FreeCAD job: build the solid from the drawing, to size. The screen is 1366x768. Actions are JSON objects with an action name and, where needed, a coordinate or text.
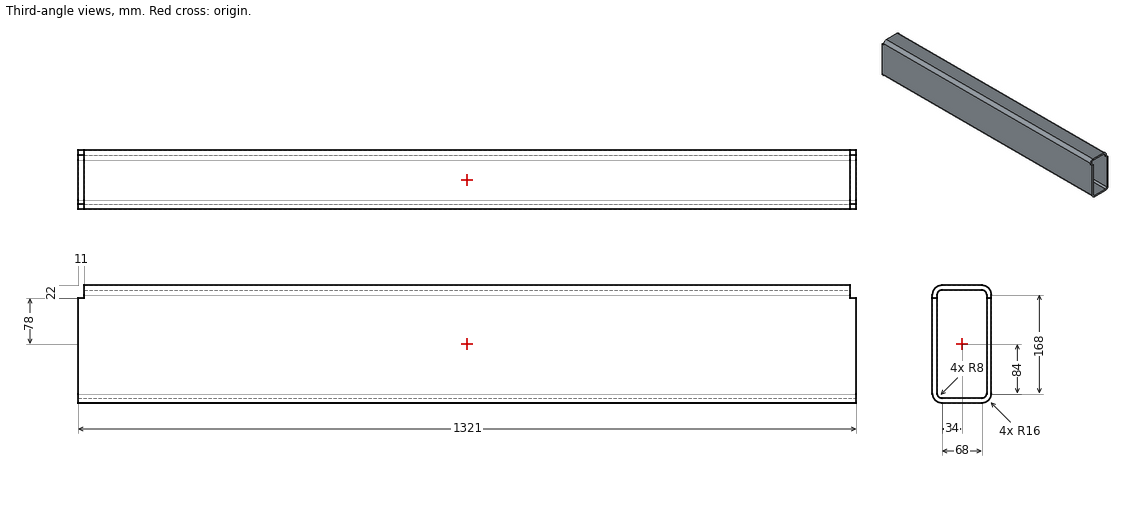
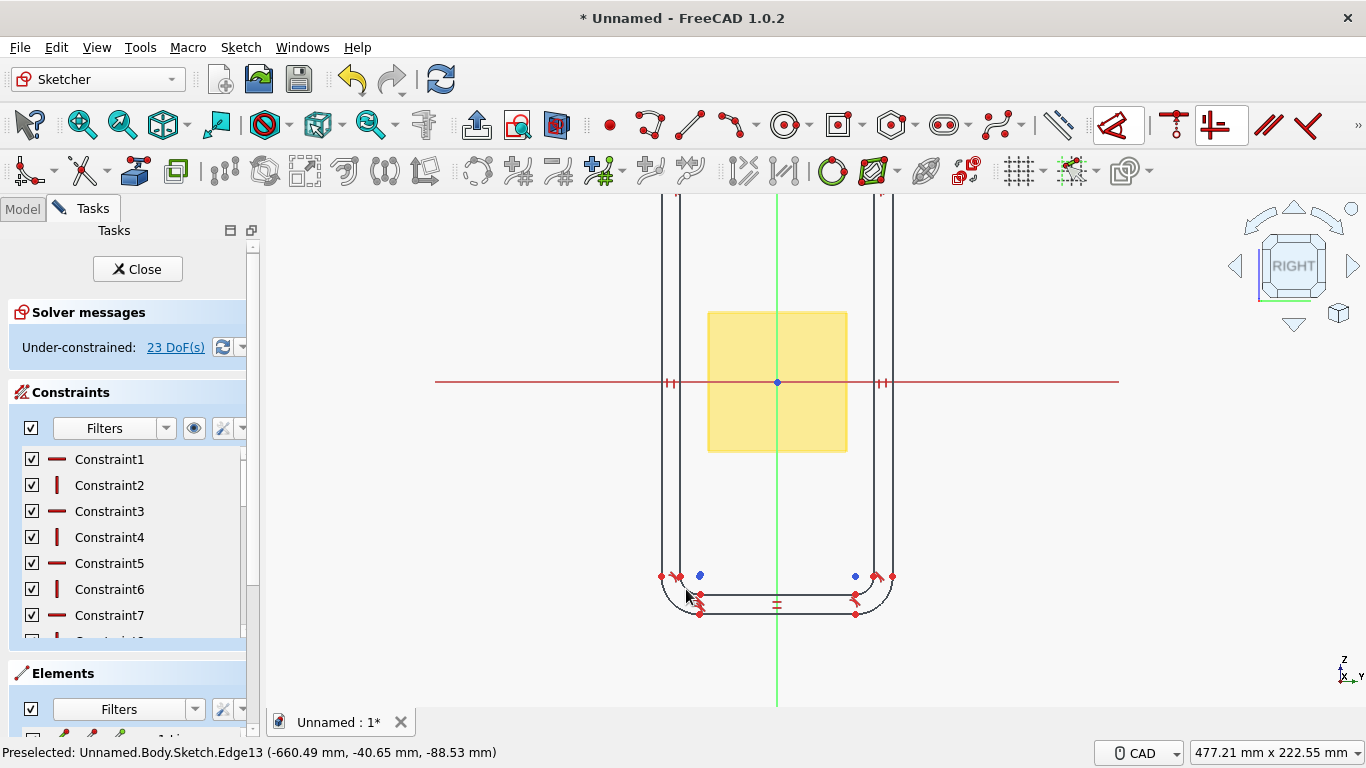
{"action": "left_click", "coordinate": [809, 595]}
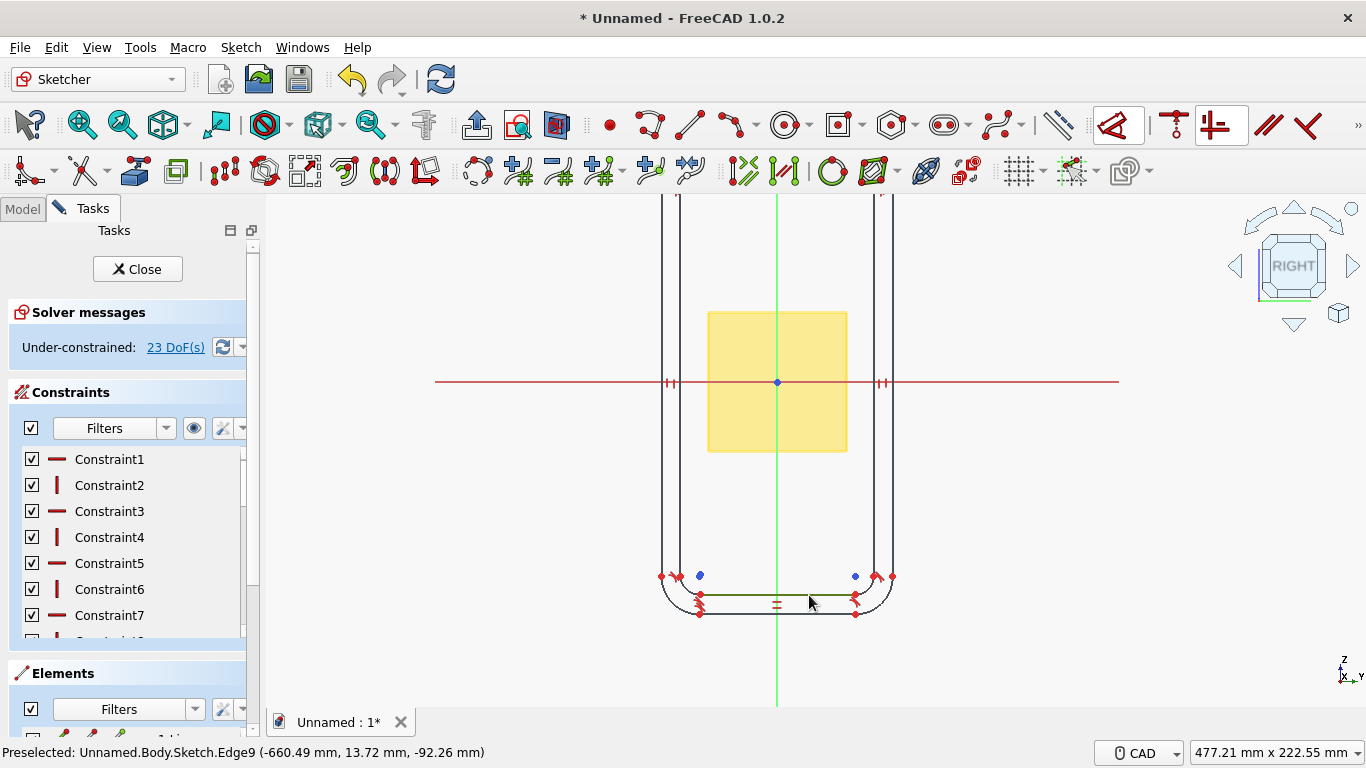
{"action": "left_click", "coordinate": [869, 589]}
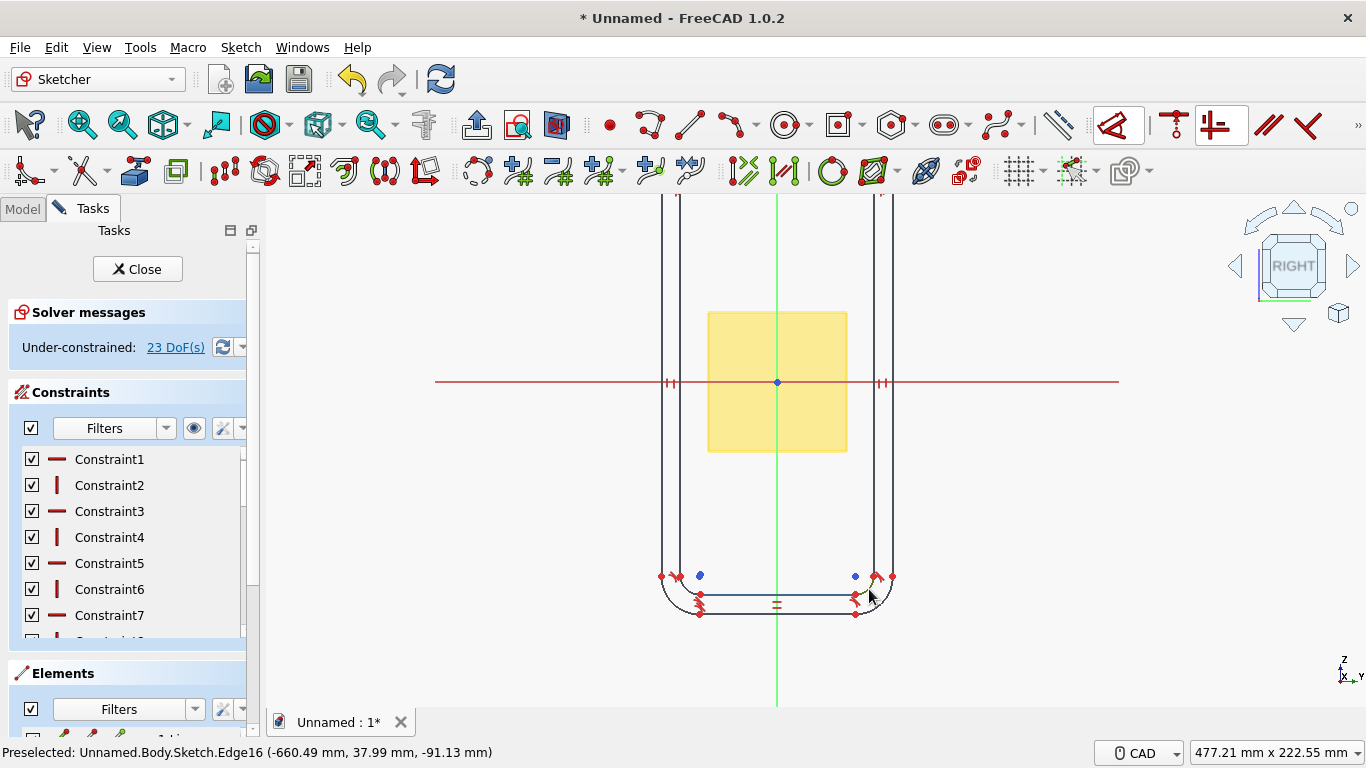
{"action": "key", "text": "t"}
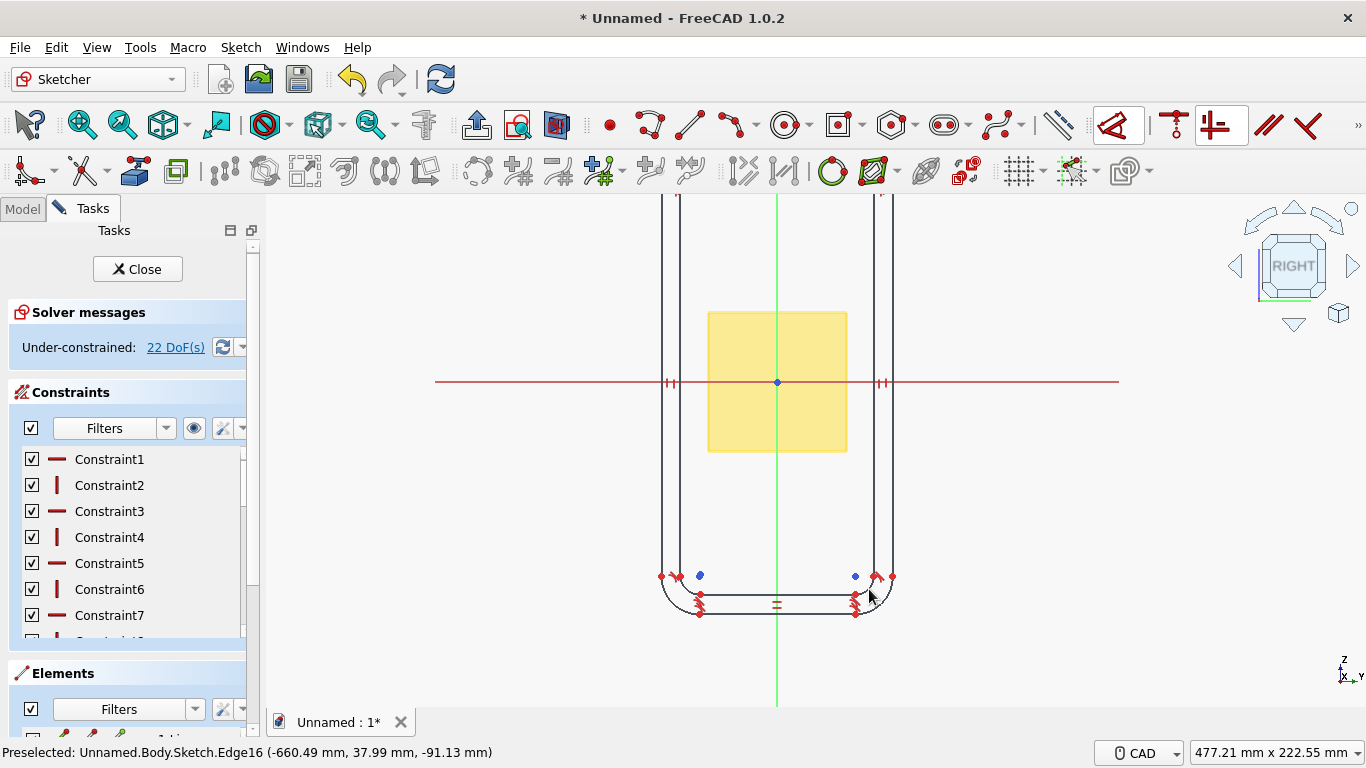
{"action": "left_click", "coordinate": [680, 460]}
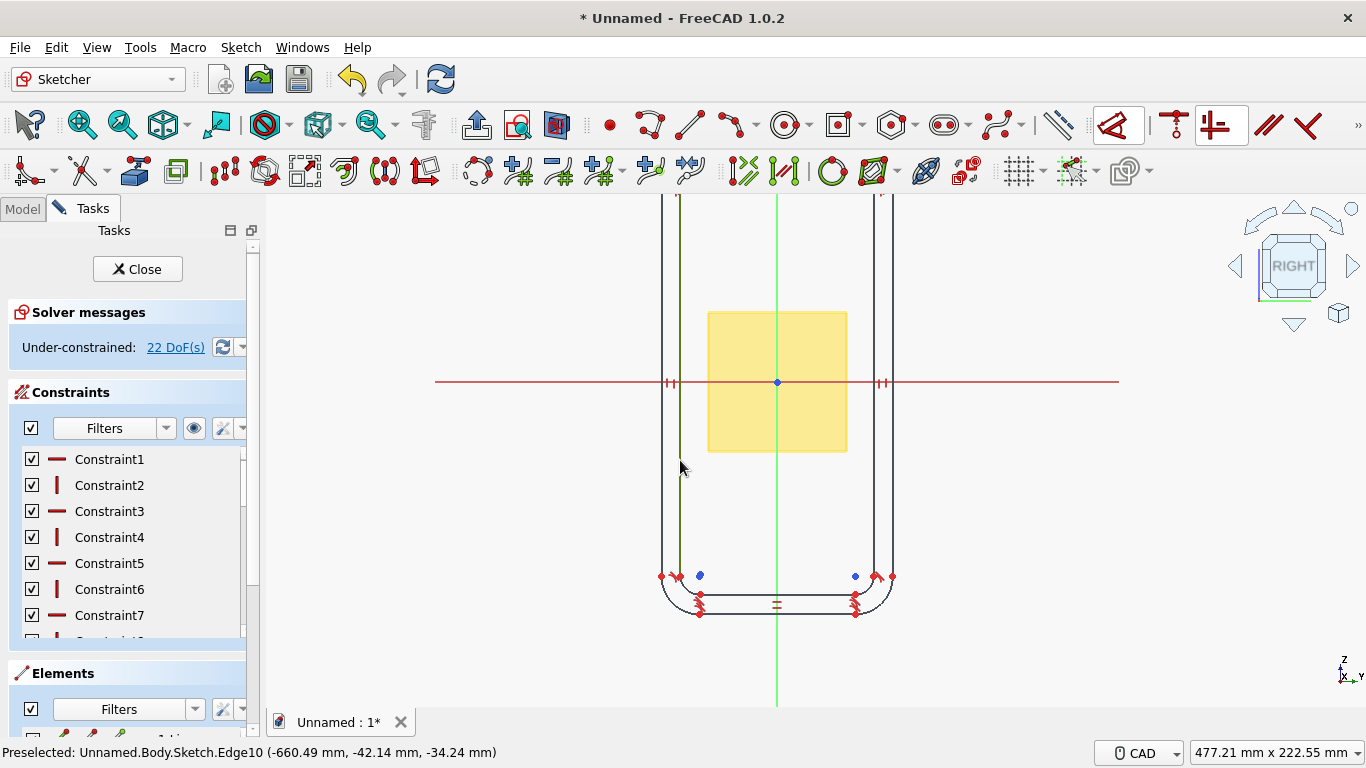
{"action": "left_click", "coordinate": [687, 590]}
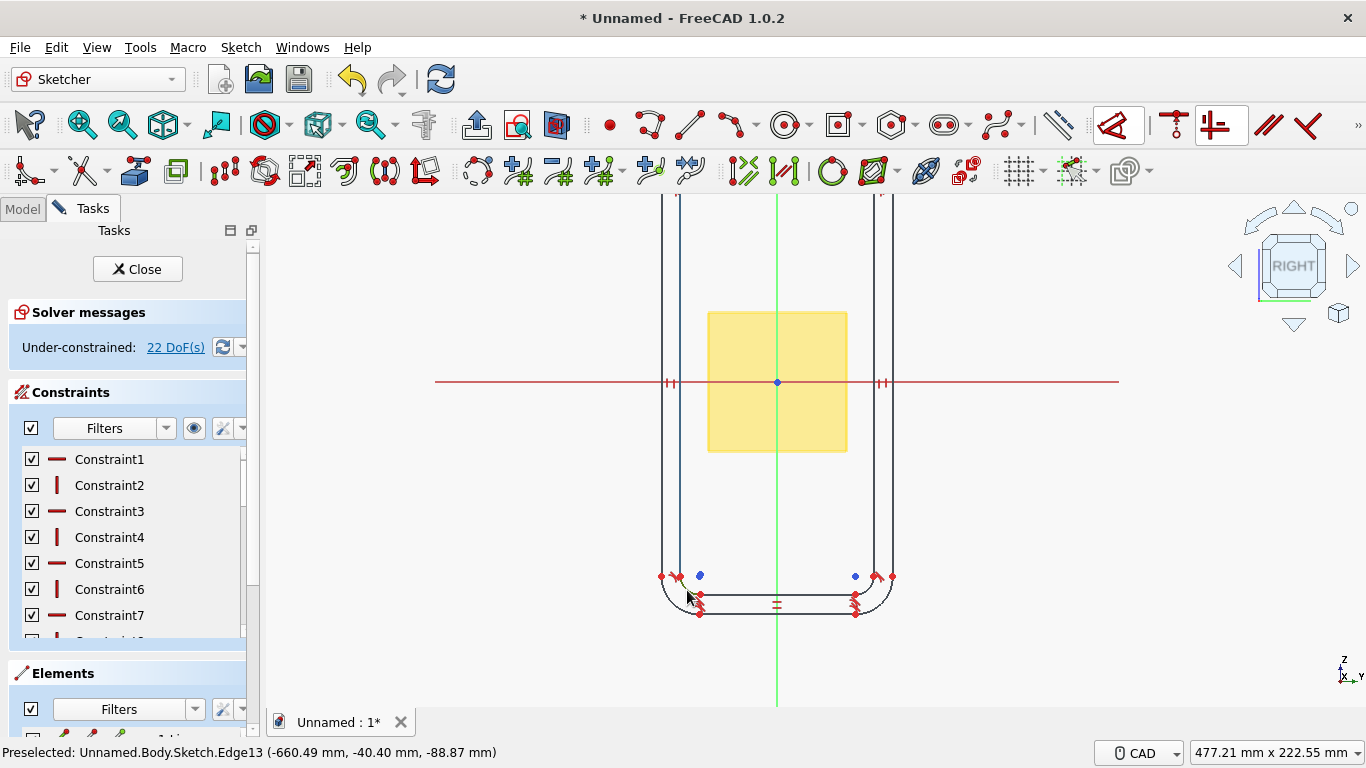
{"action": "key", "text": "t"}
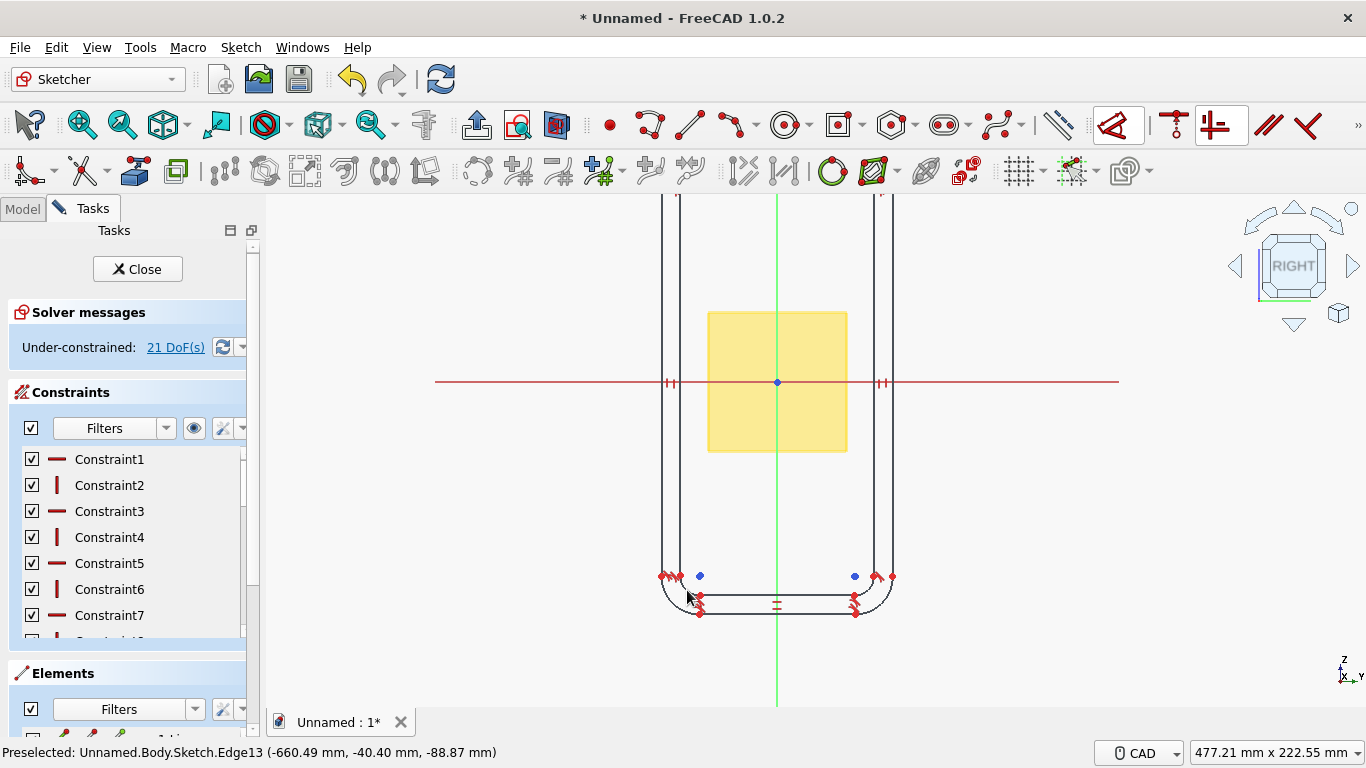
{"action": "left_click", "coordinate": [680, 460]}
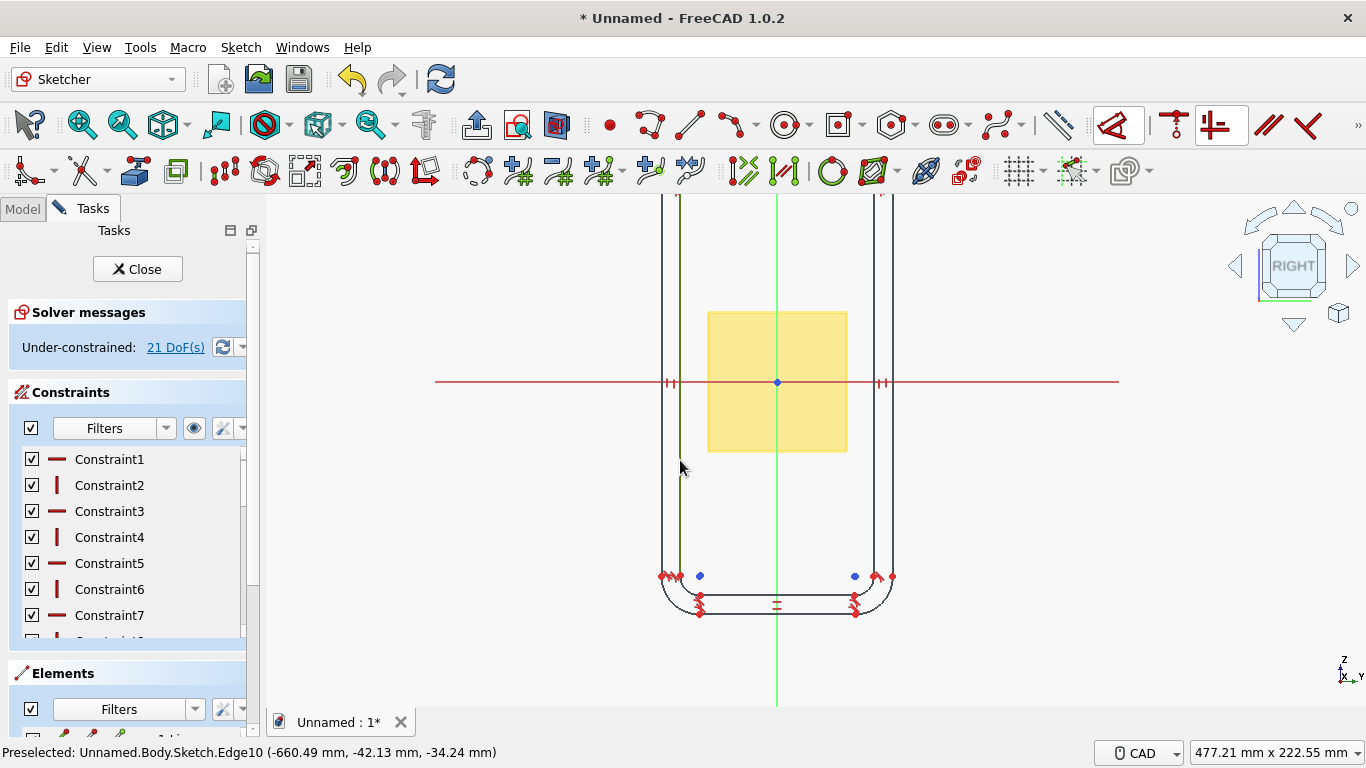
{"action": "scroll", "coordinate": [687, 590], "scroll_direction": "down", "scroll_amount": 2}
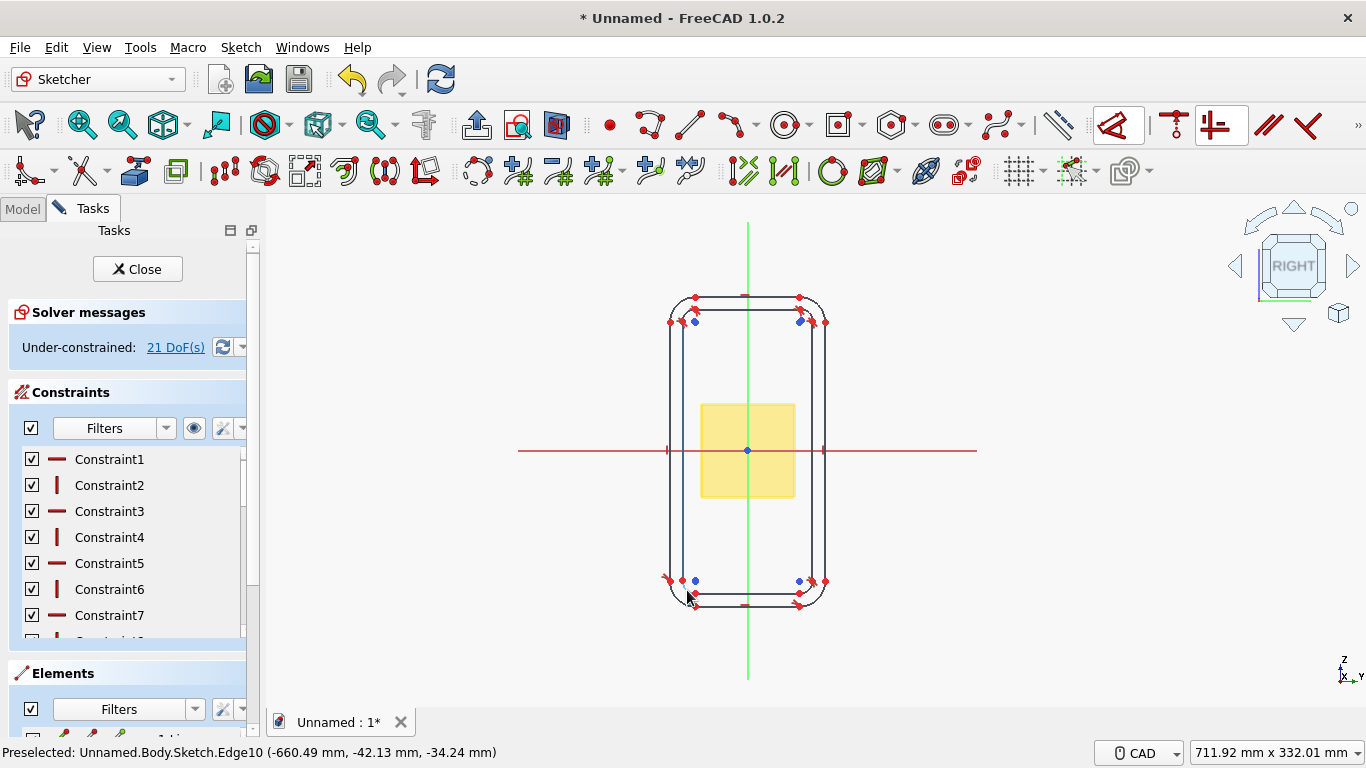
{"action": "scroll", "coordinate": [686, 313], "scroll_direction": "up", "scroll_amount": 2}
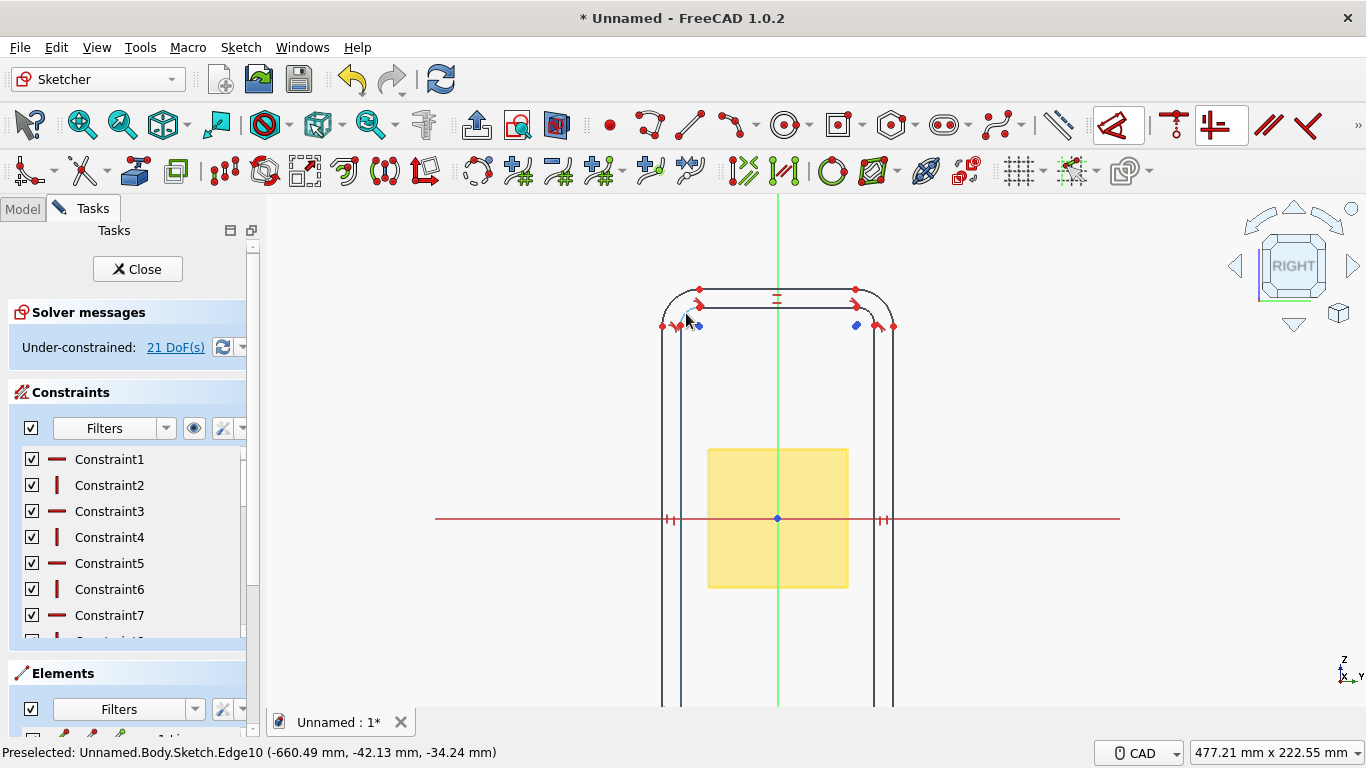
{"action": "left_click", "coordinate": [686, 313]}